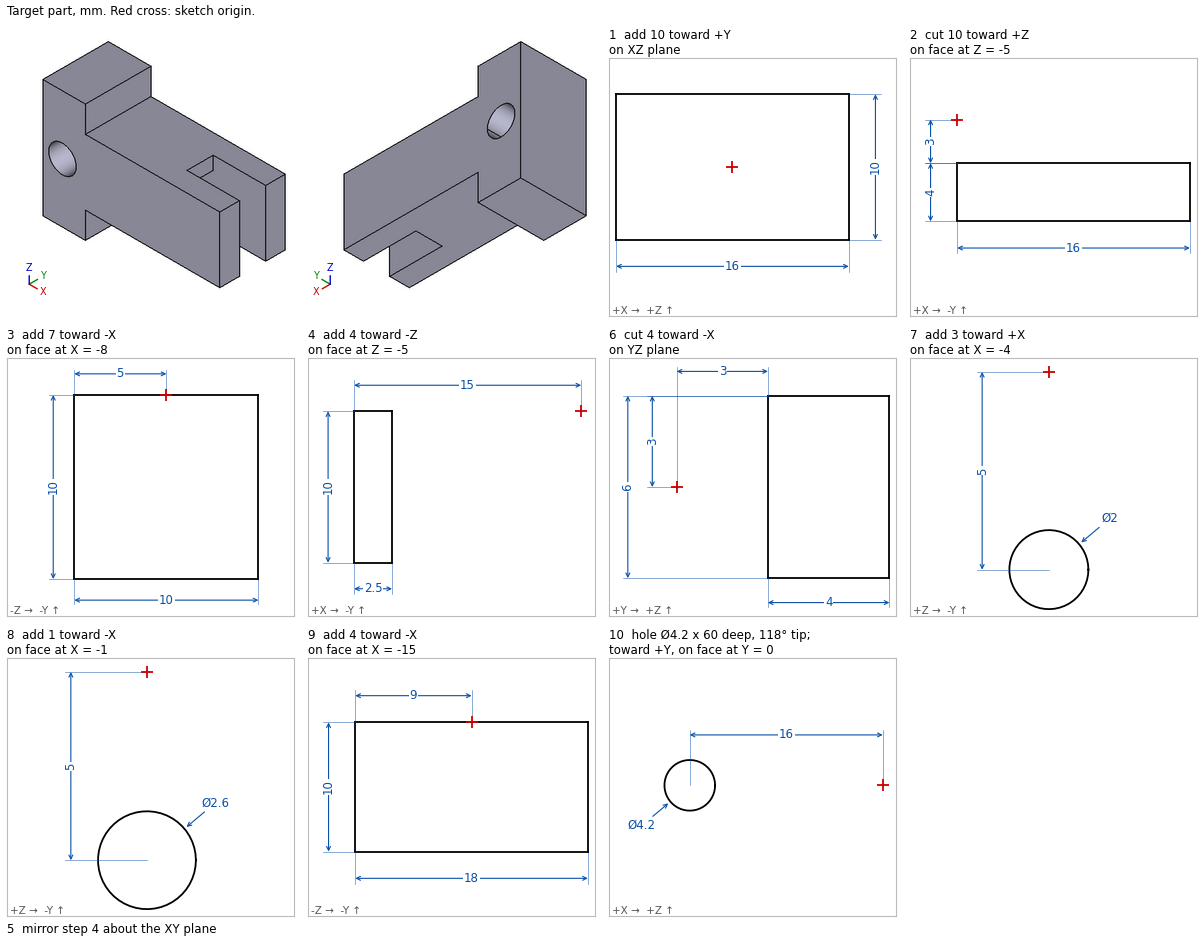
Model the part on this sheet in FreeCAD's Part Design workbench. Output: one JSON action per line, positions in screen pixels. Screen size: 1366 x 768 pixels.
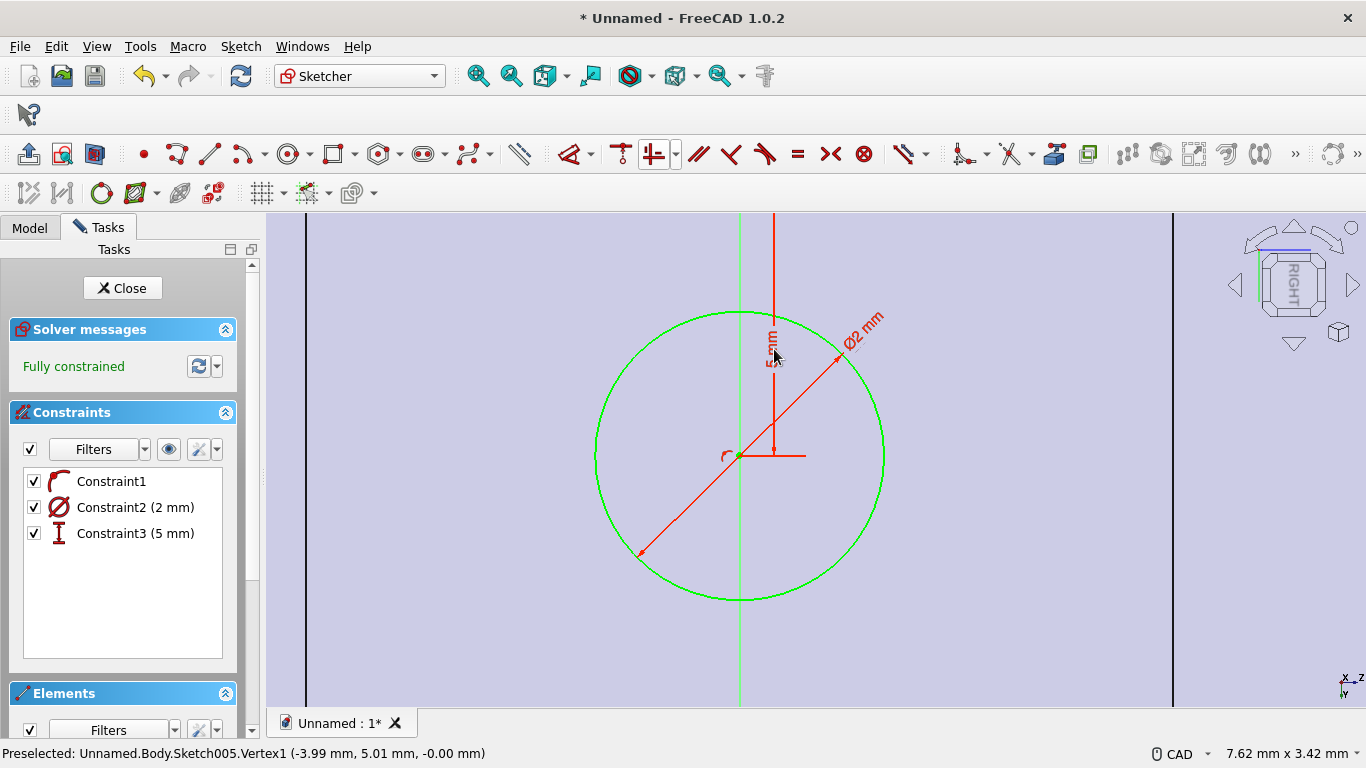
{"action": "left_click", "coordinate": [123, 288]}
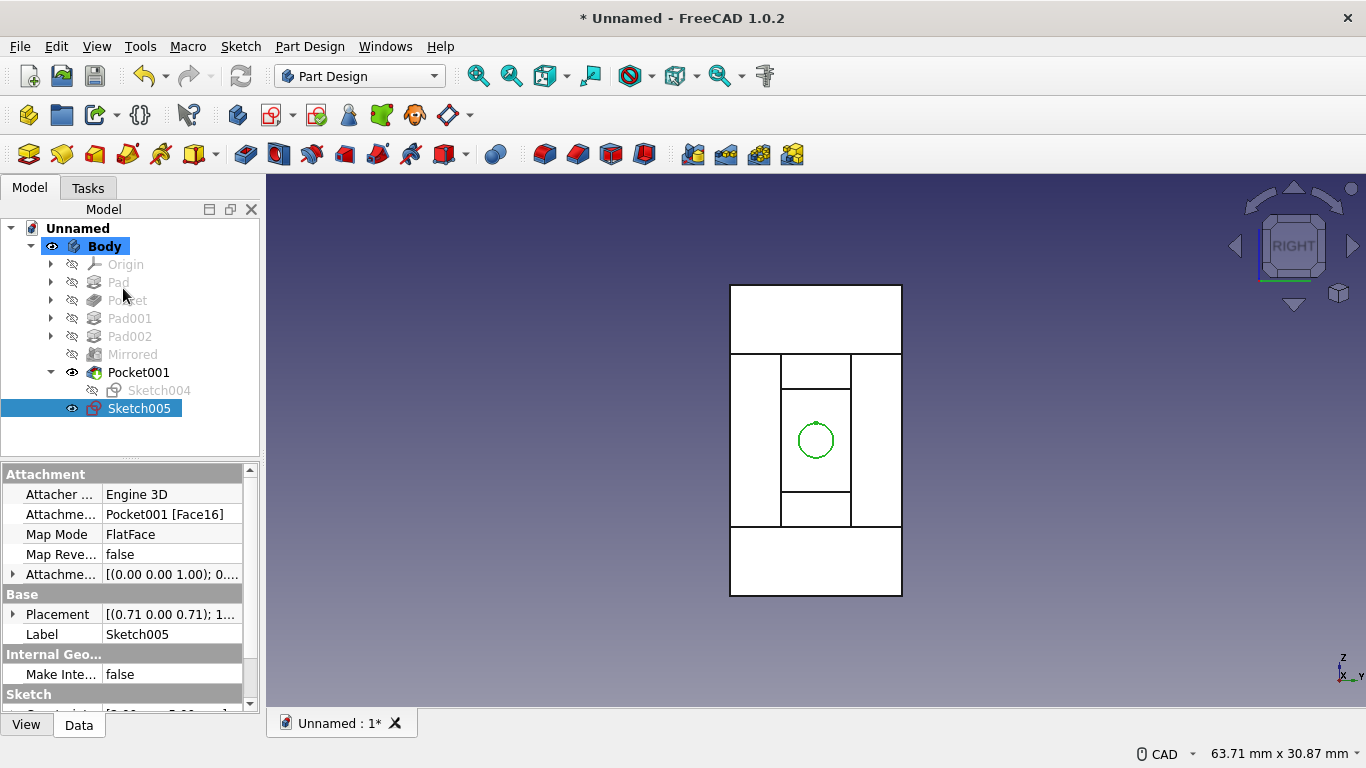
{"action": "left_click", "coordinate": [29, 154]}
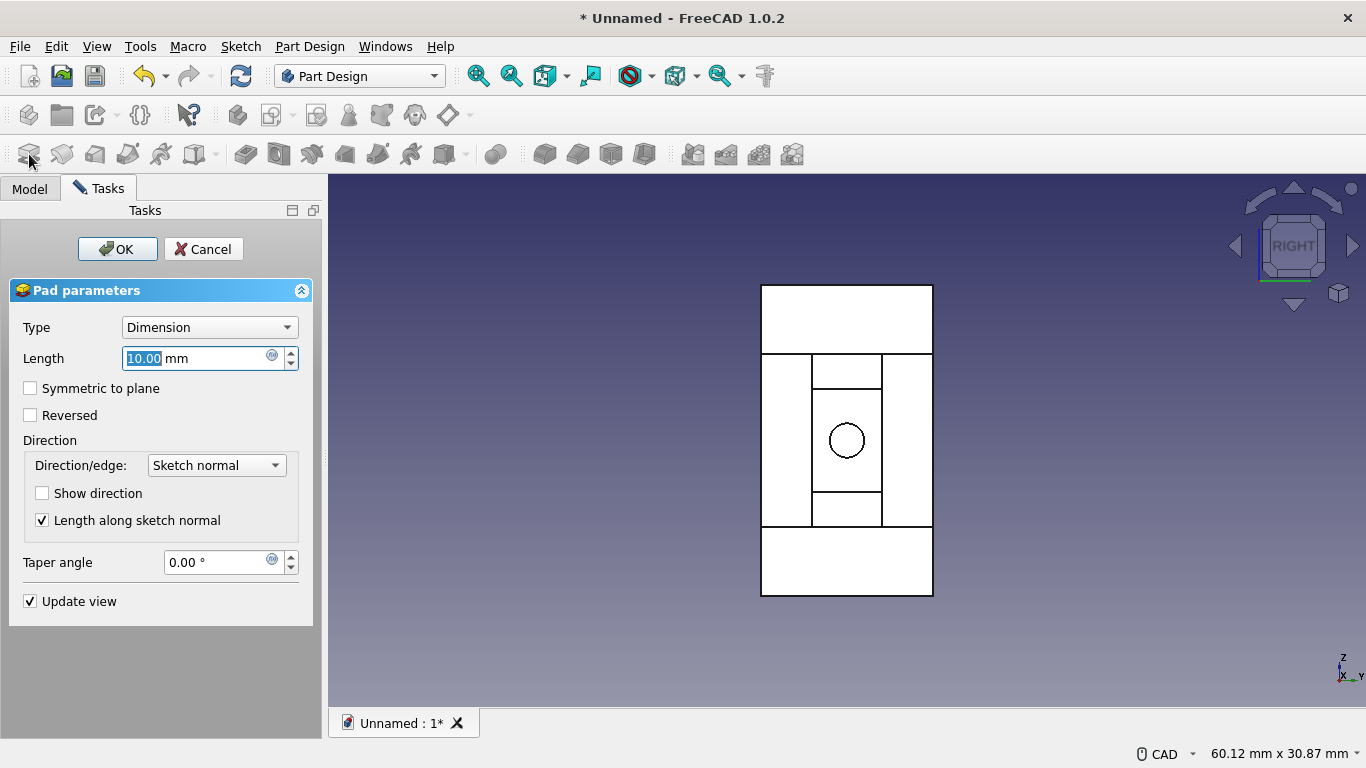
{"action": "type", "text": "3"}
{"action": "key", "text": "Tab"}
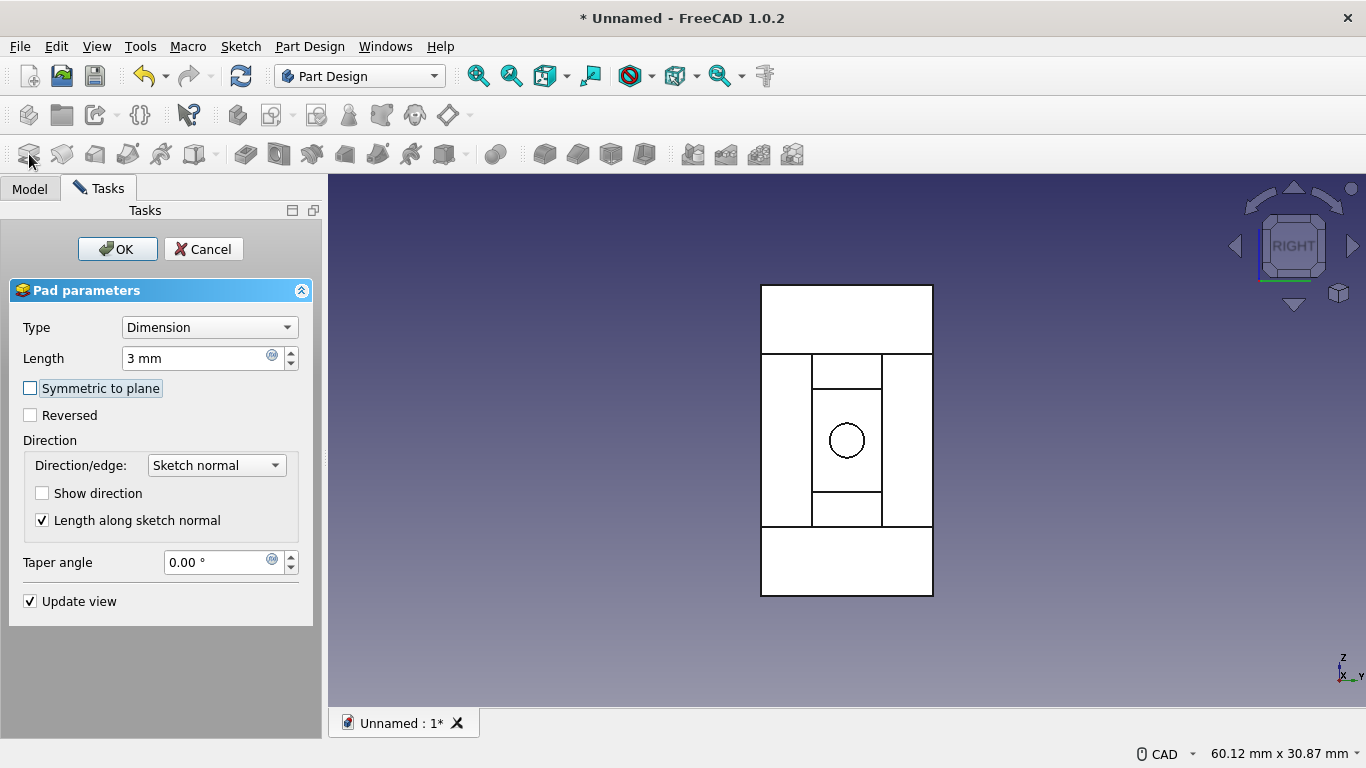
{"action": "left_click", "coordinate": [118, 249]}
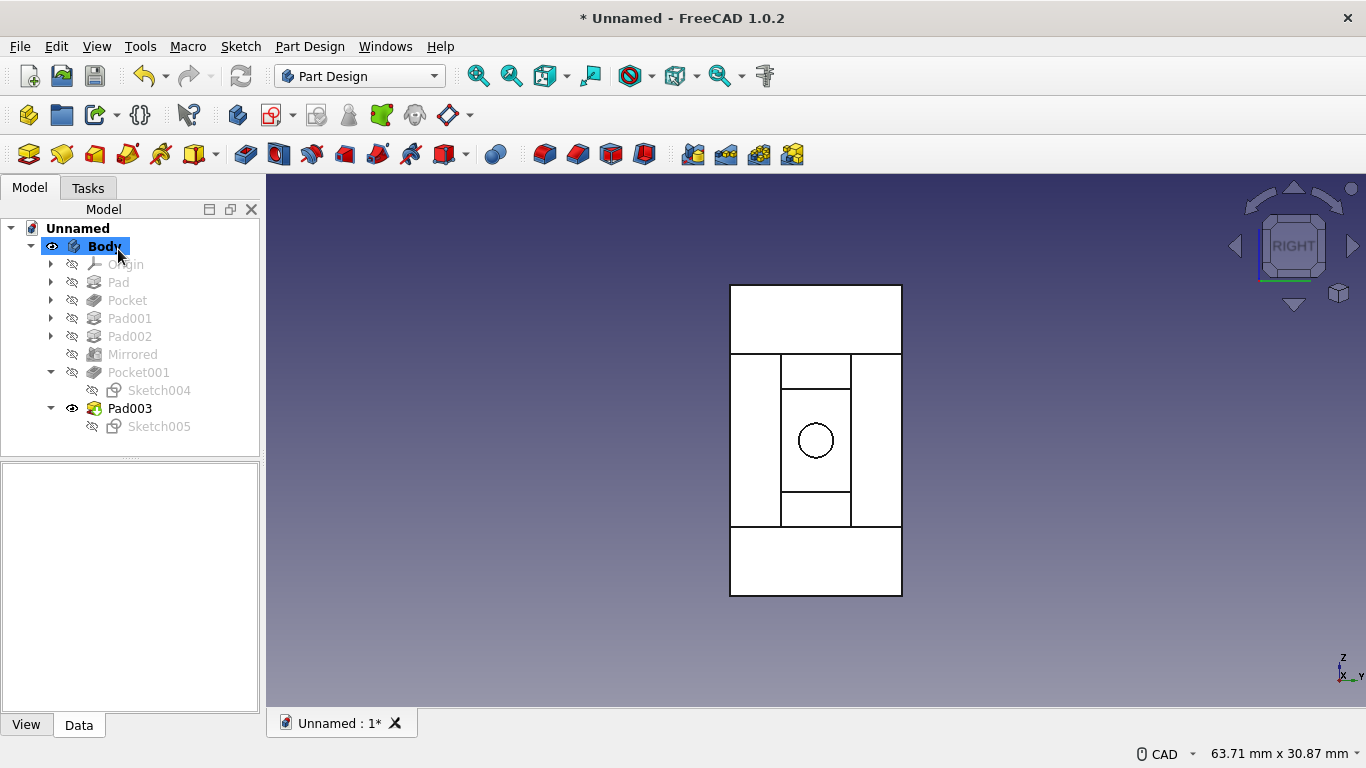
{"action": "left_click", "coordinate": [816, 440]}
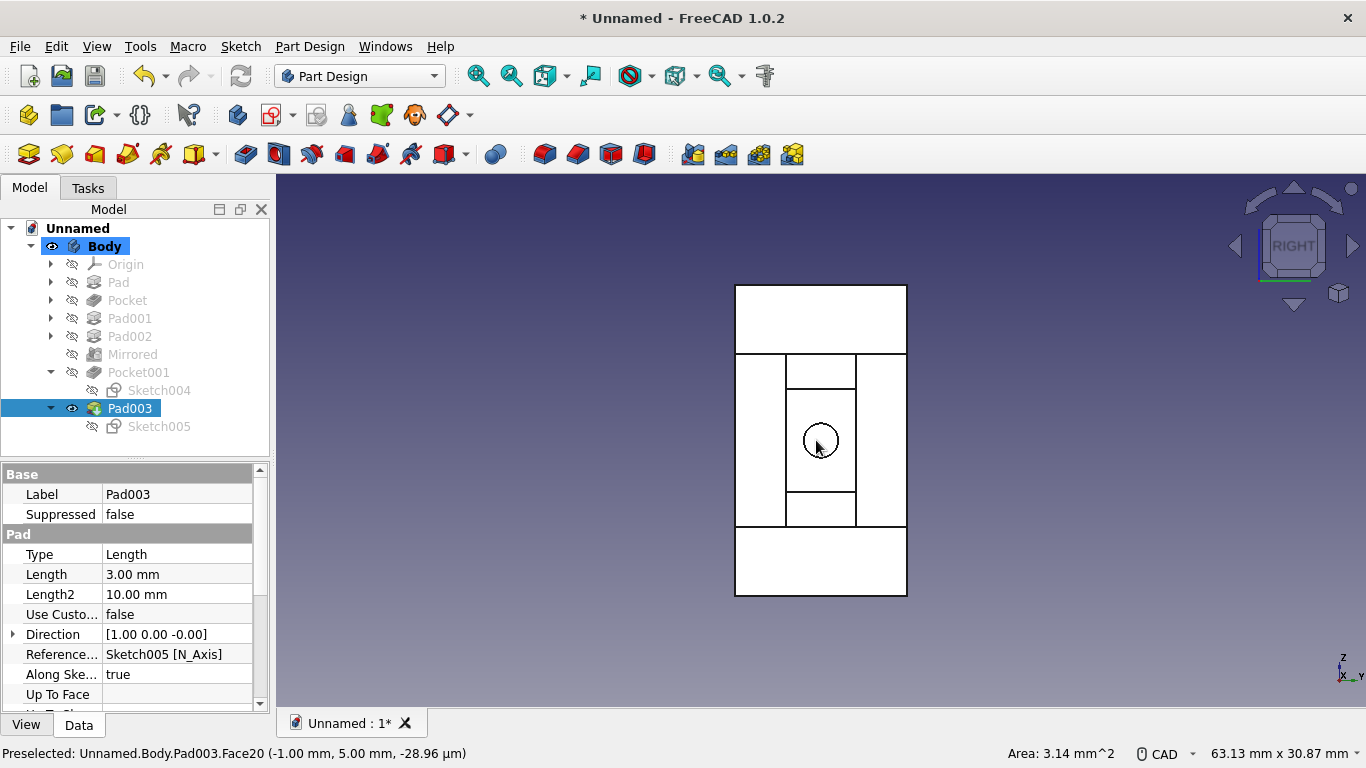
{"action": "left_click", "coordinate": [270, 116]}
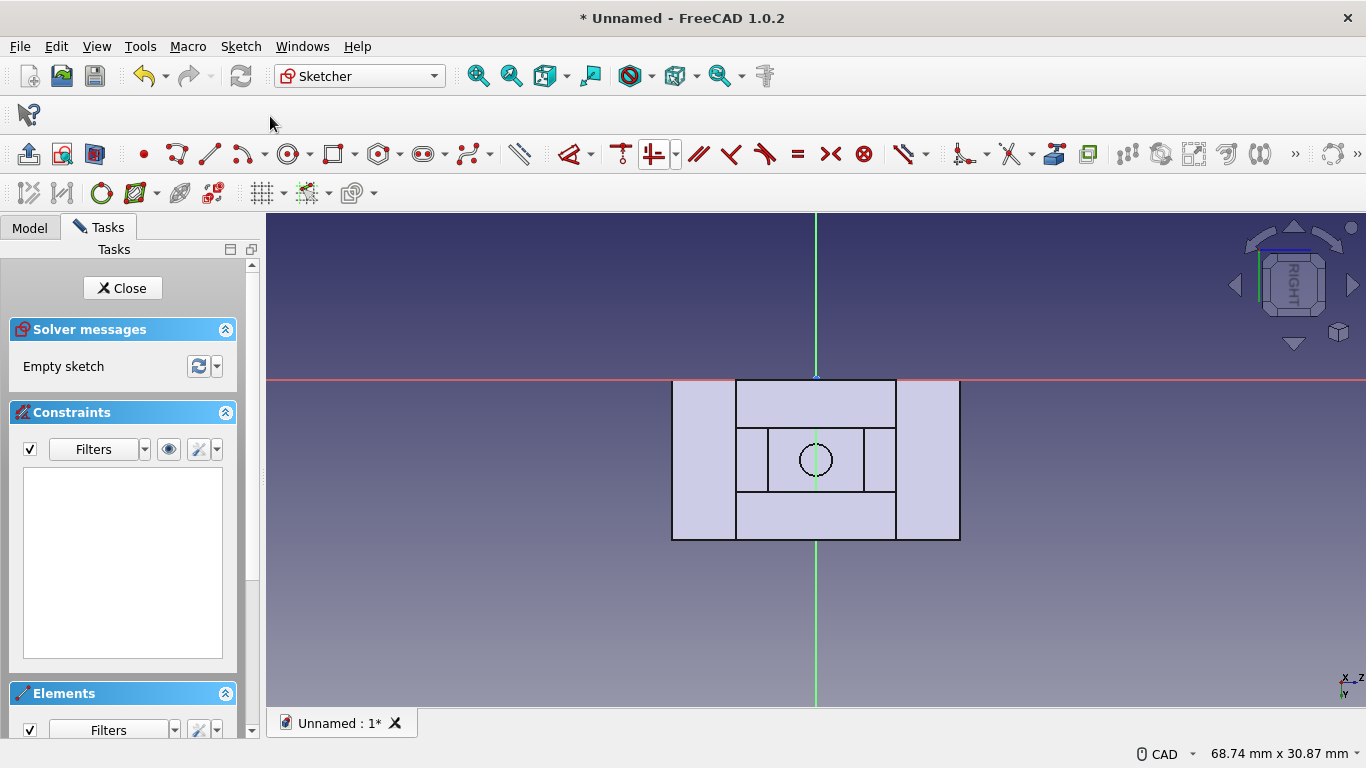
{"action": "left_click", "coordinate": [95, 154]}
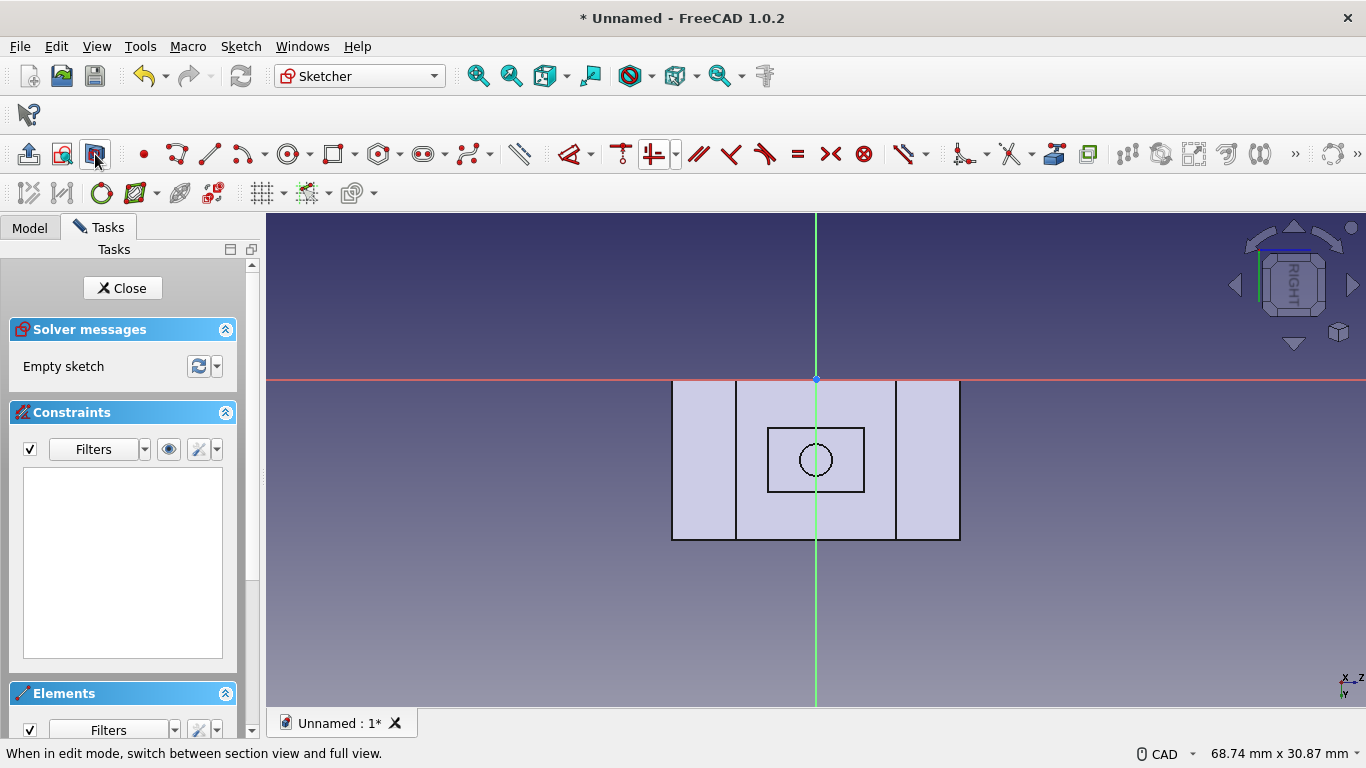
{"action": "scroll", "coordinate": [846, 418], "scroll_direction": "up", "scroll_amount": 6}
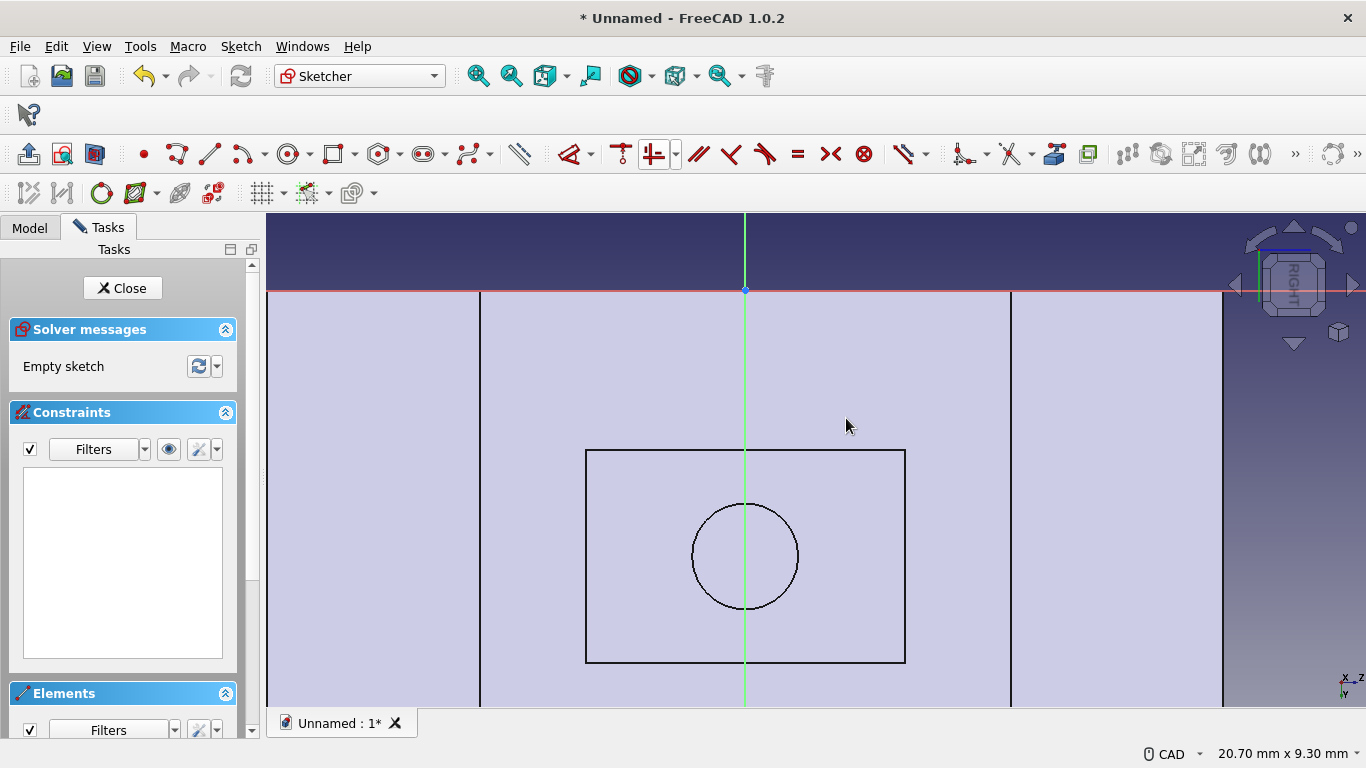
{"action": "left_click", "coordinate": [288, 154]}